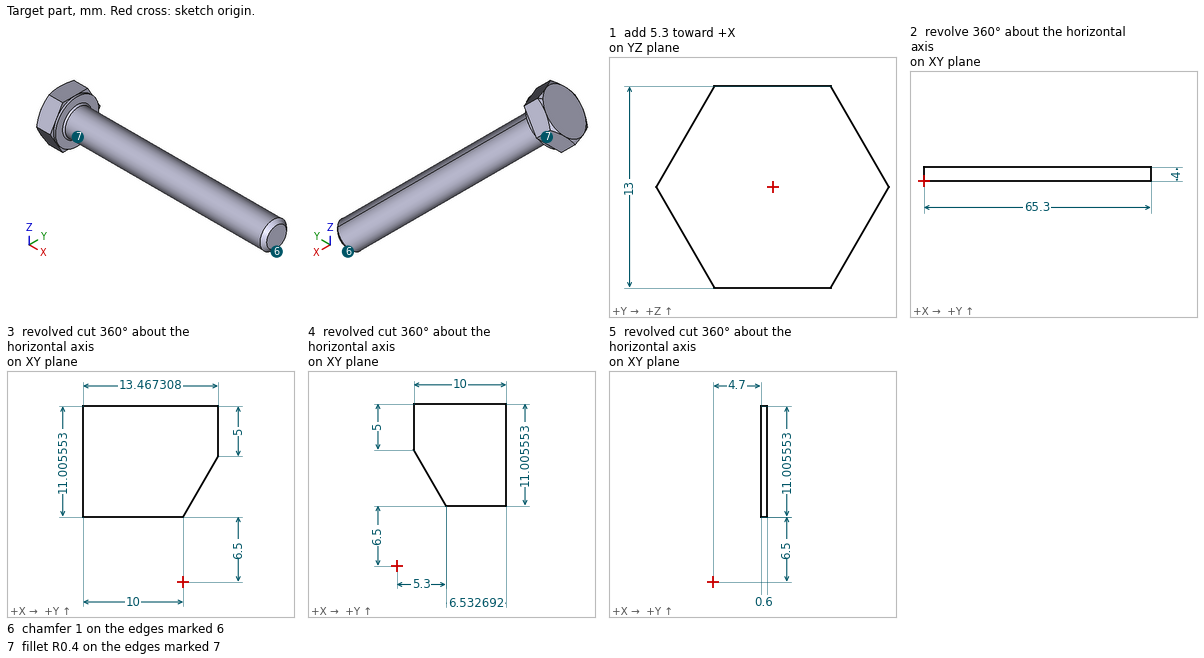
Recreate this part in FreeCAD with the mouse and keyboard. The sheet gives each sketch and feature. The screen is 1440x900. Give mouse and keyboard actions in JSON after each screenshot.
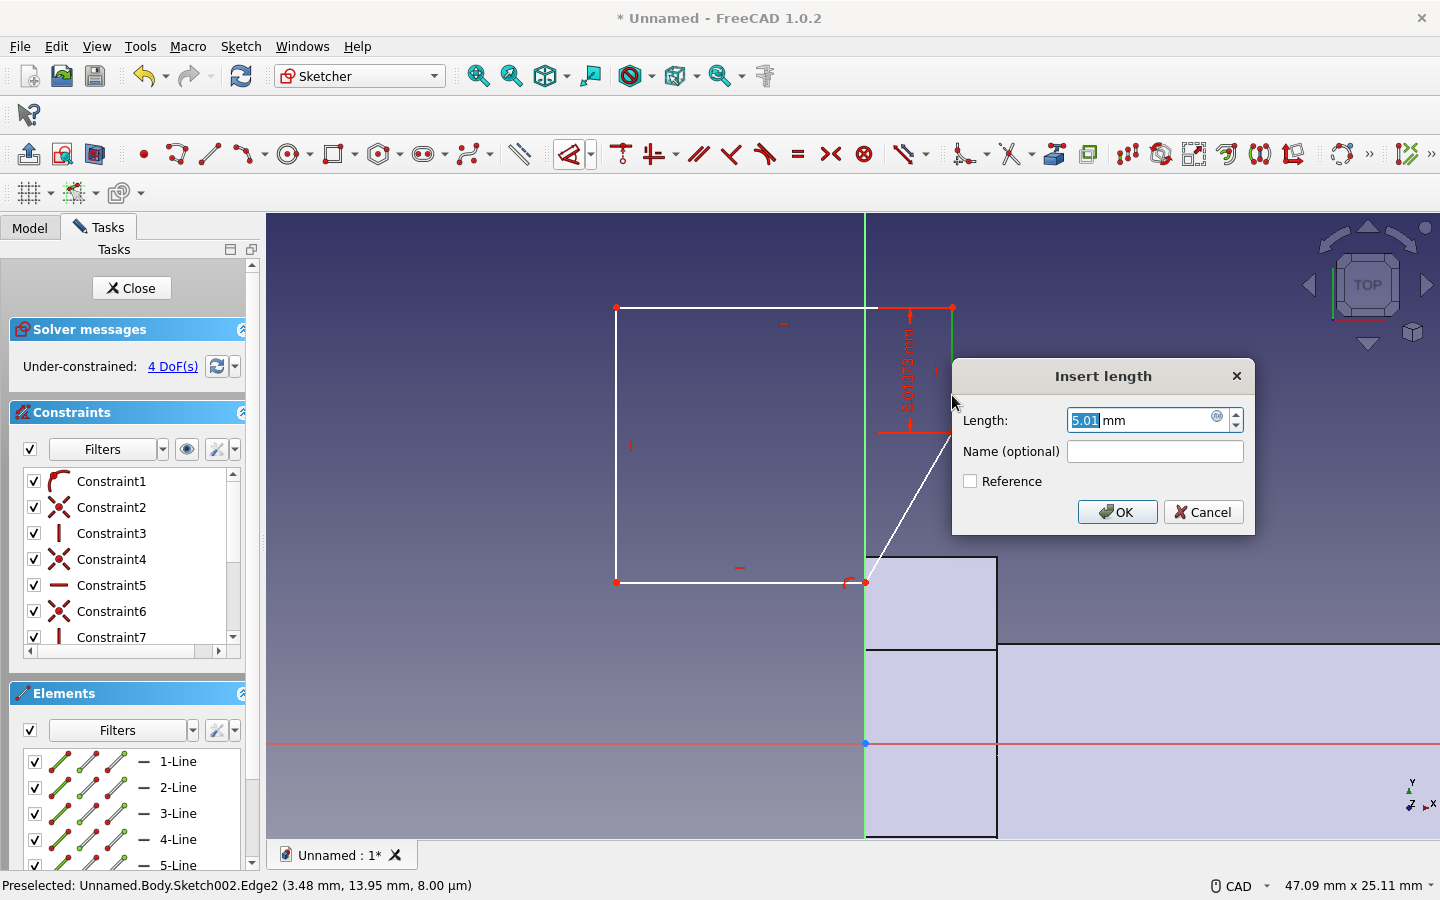
{"action": "type", "text": "5"}
{"action": "key", "text": "Return"}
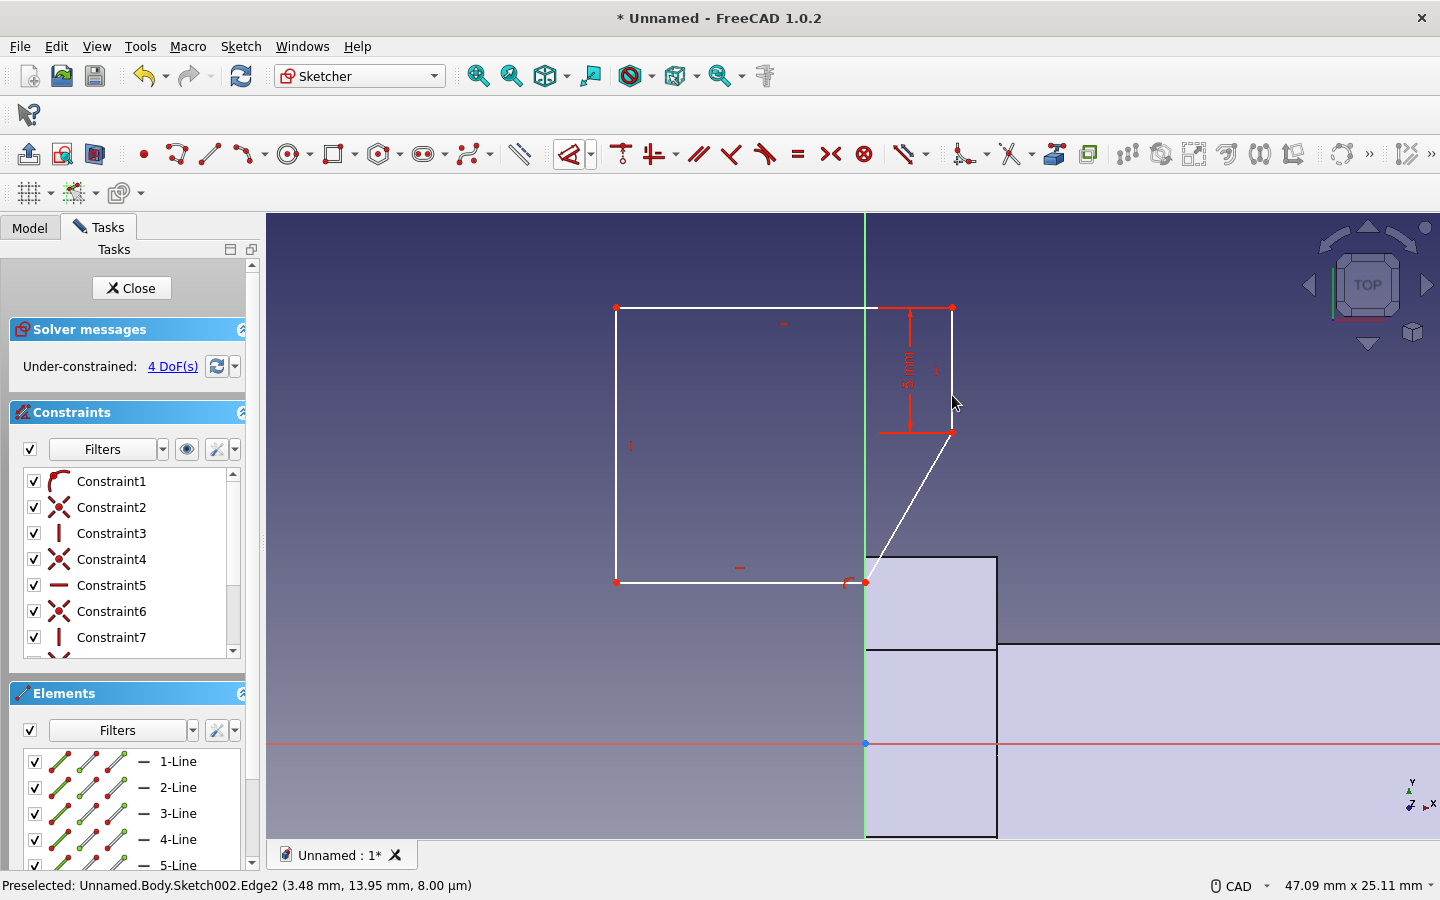
{"action": "left_click", "coordinate": [691, 583]}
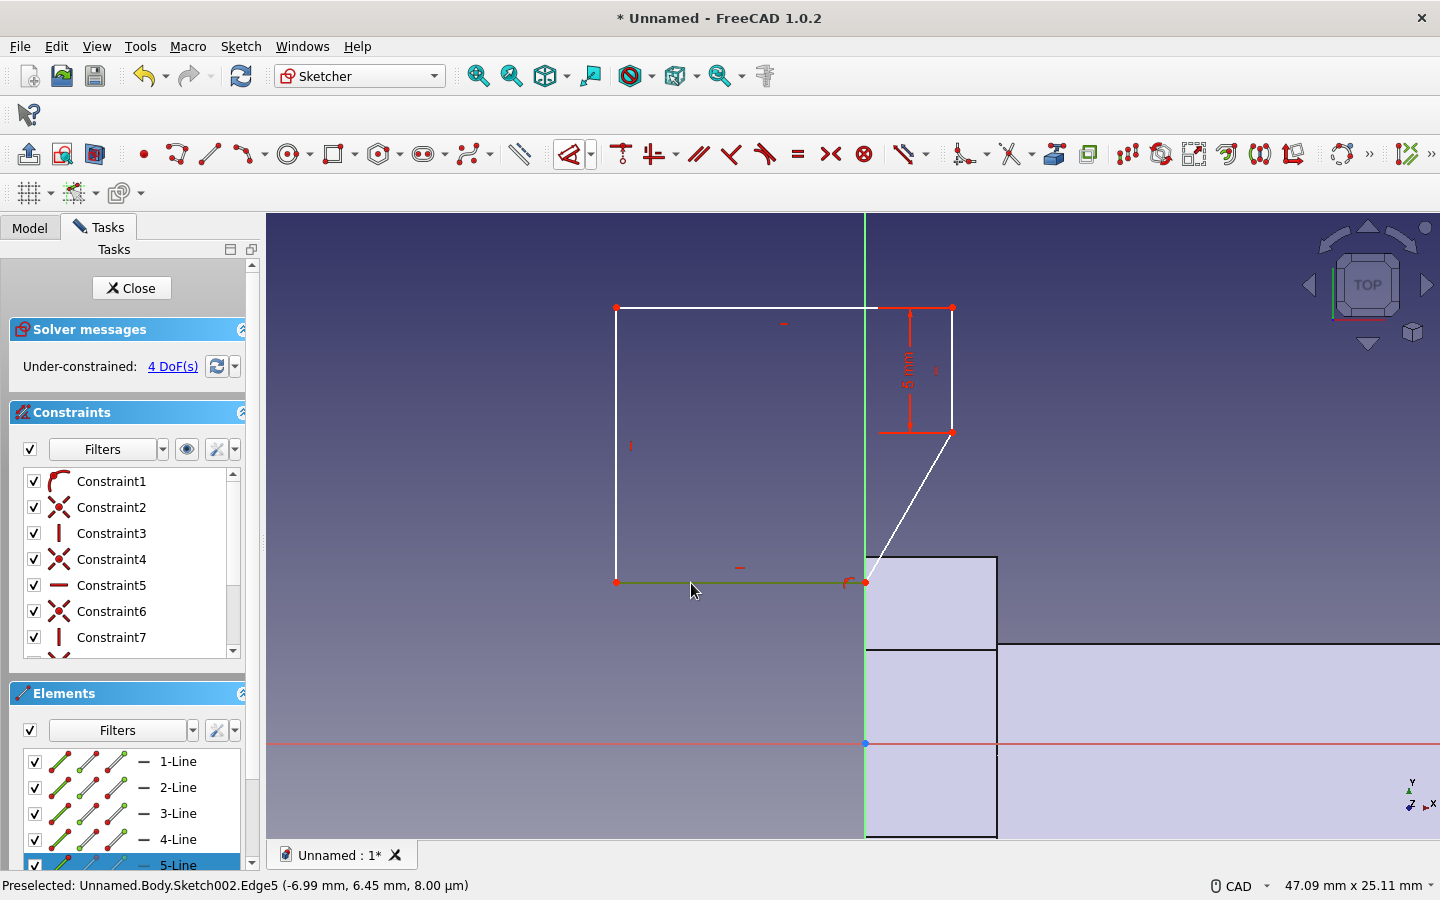
{"action": "left_click", "coordinate": [590, 154]}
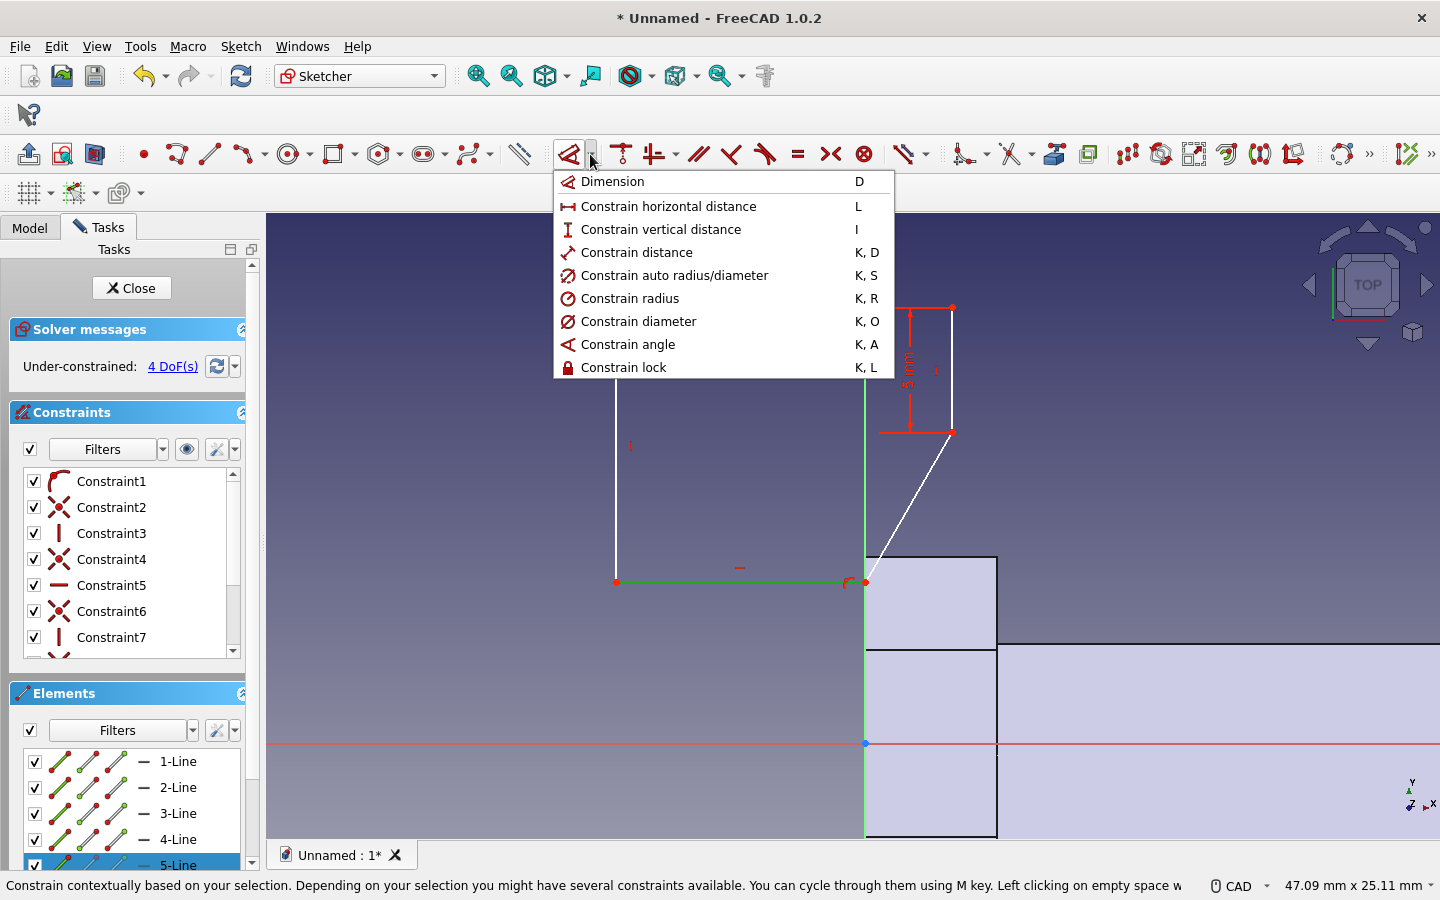
{"action": "left_click", "coordinate": [724, 206]}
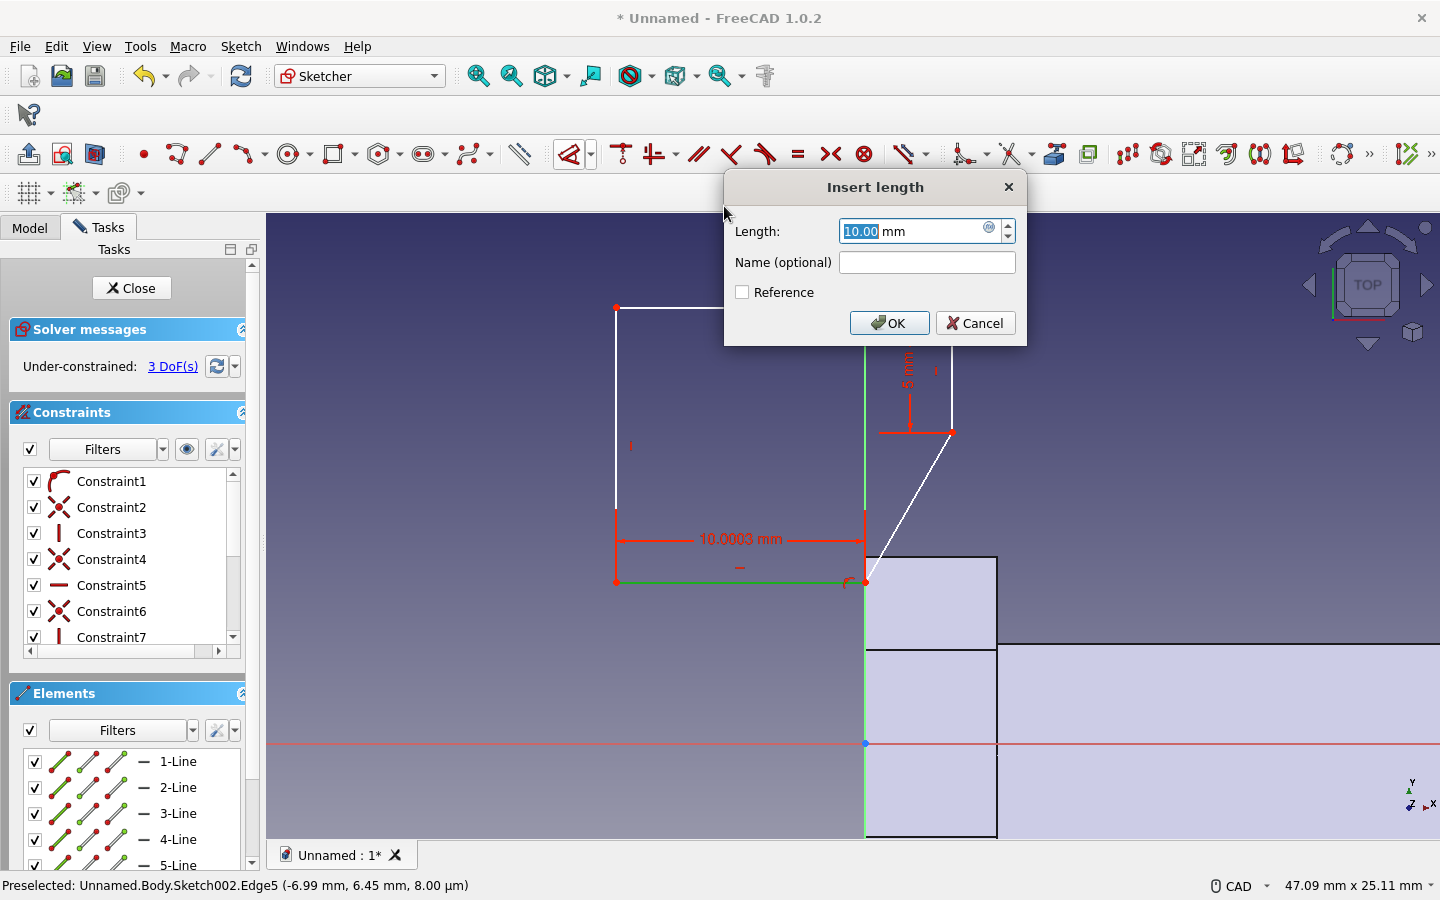
{"action": "type", "text": "10"}
{"action": "key", "text": "Return"}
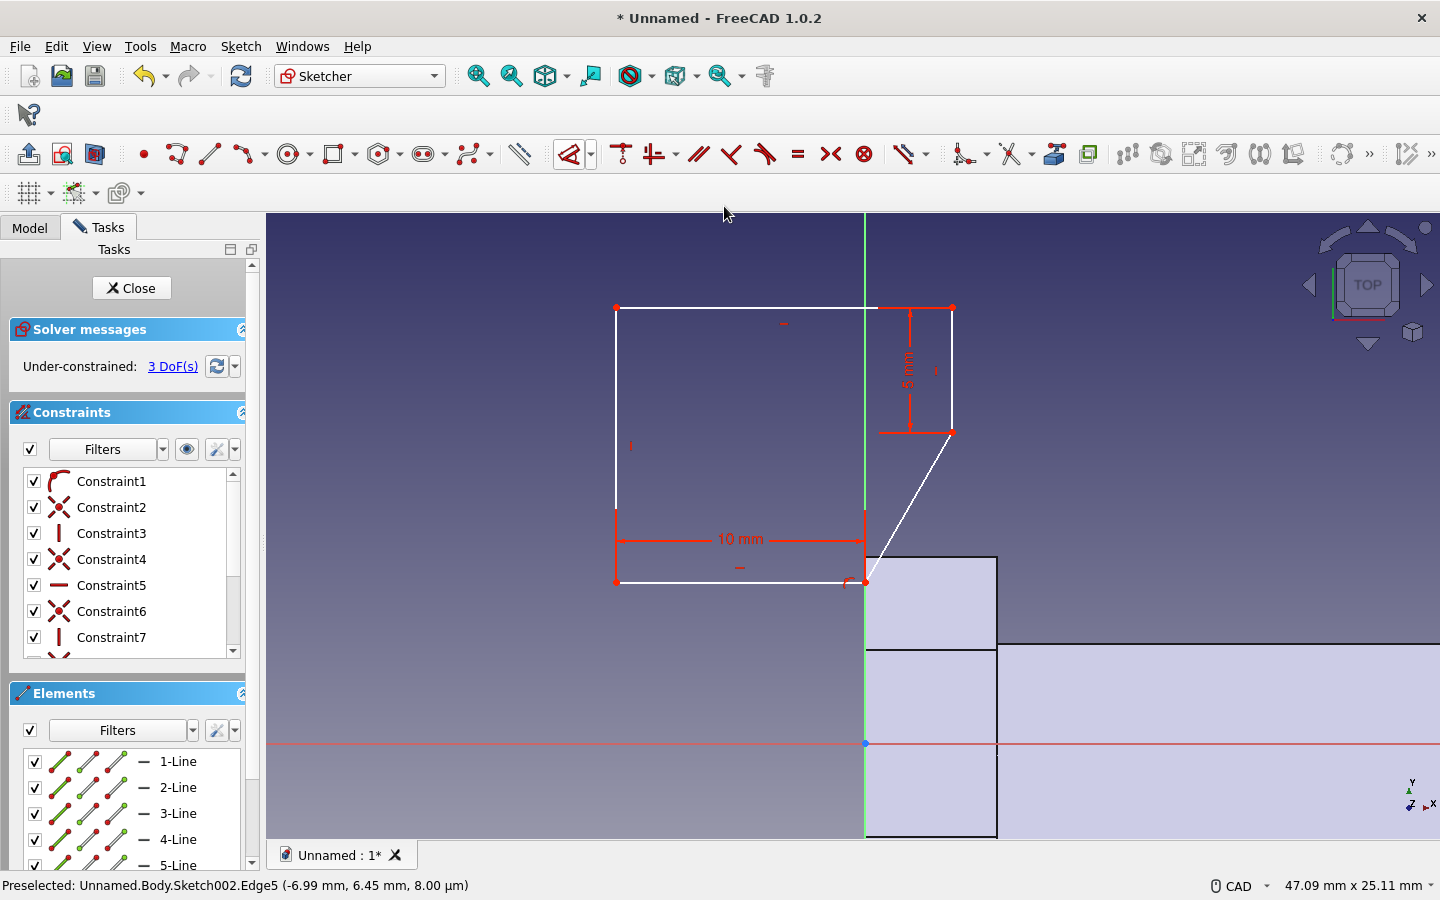
{"action": "left_click", "coordinate": [865, 583]}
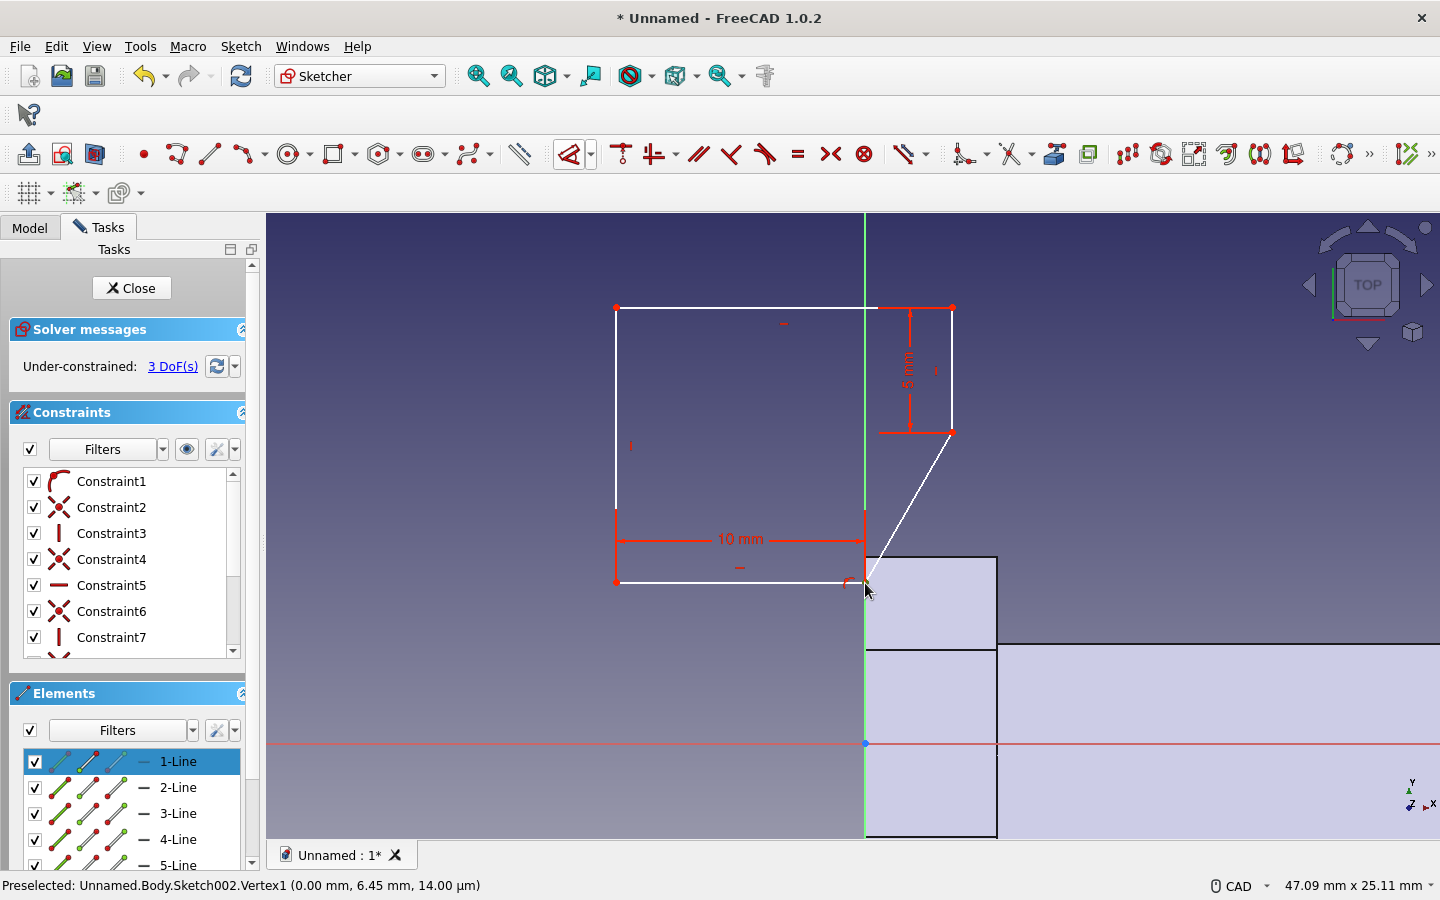
{"action": "left_click", "coordinate": [590, 154]}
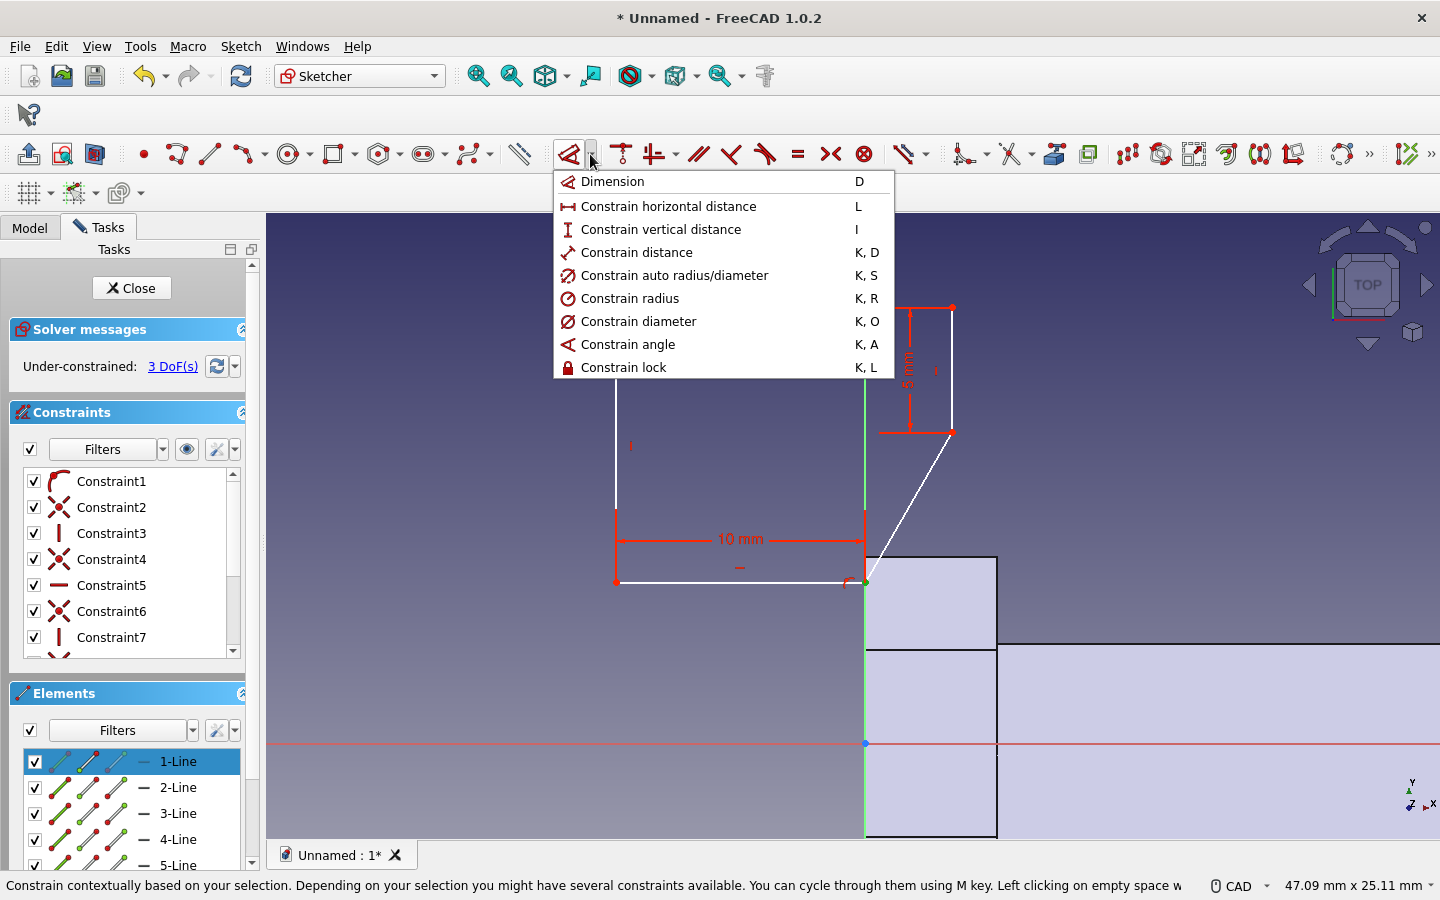
{"action": "left_click", "coordinate": [724, 230]}